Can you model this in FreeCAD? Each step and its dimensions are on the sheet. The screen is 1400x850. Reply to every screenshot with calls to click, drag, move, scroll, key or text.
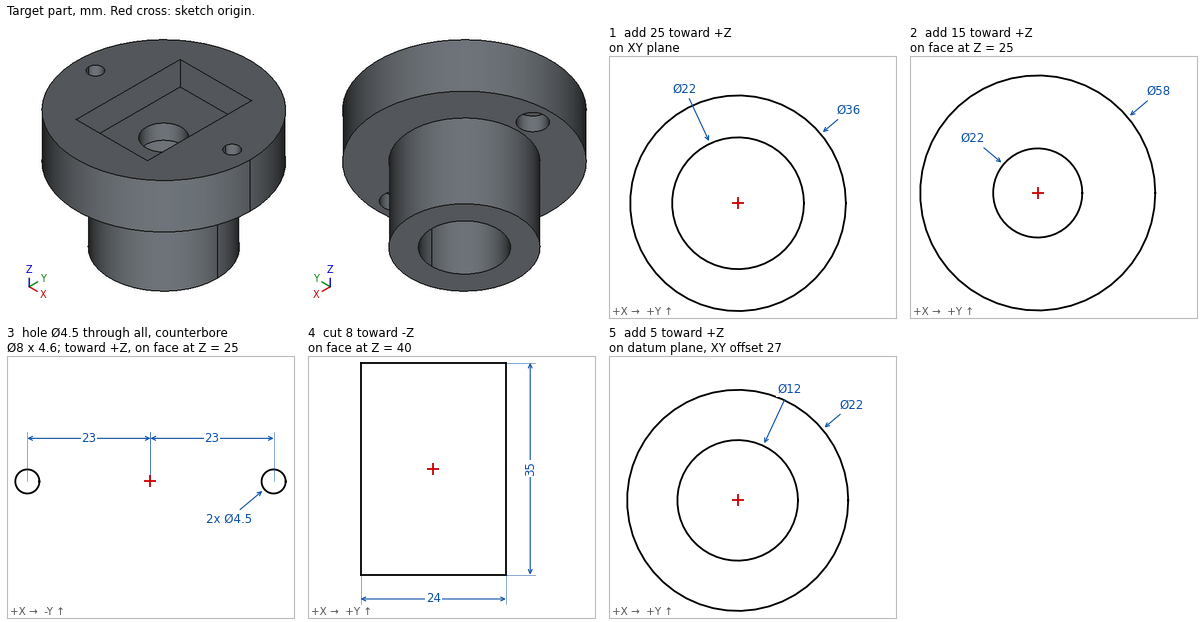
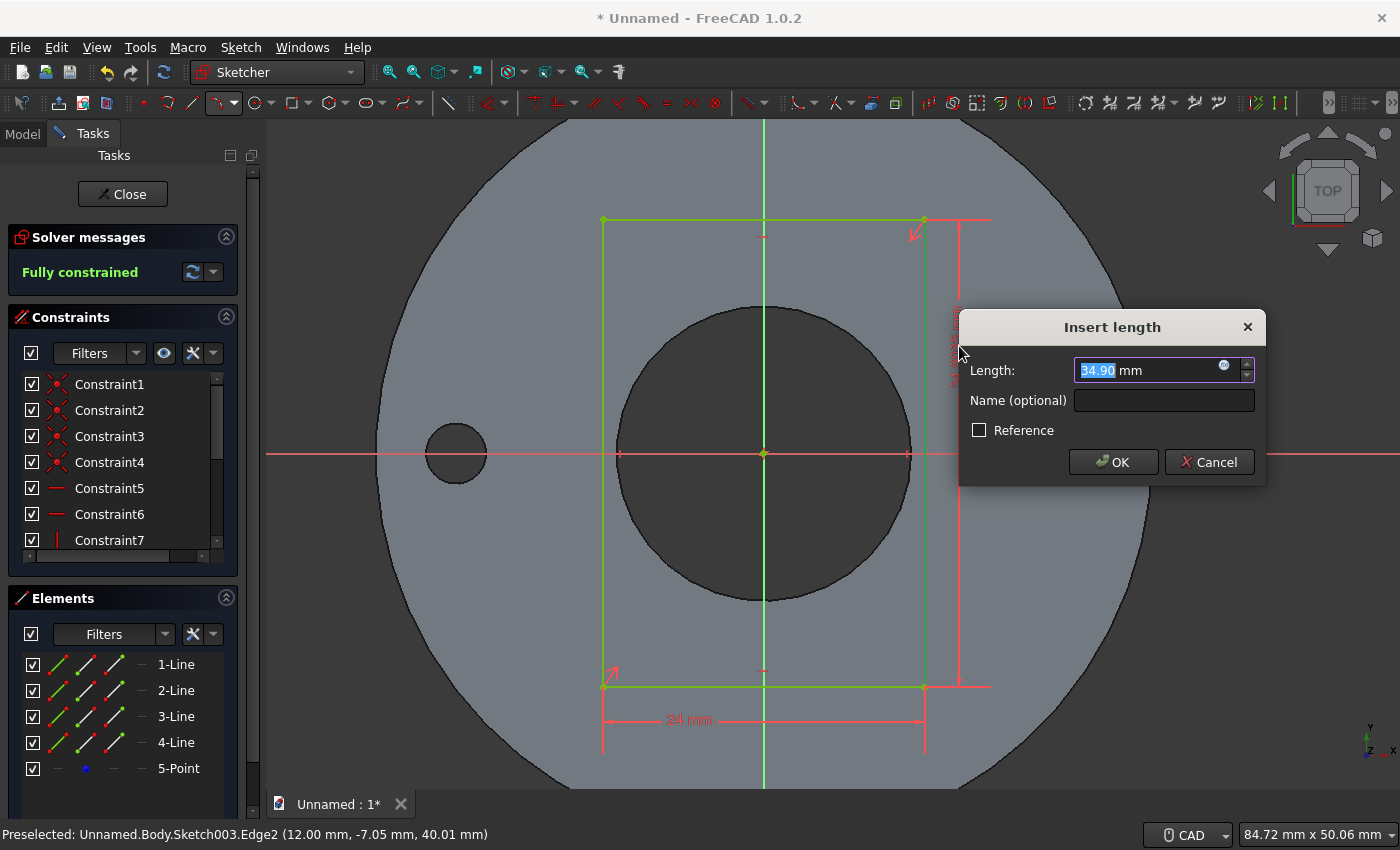
text(35)
key(Return)
key(Escape)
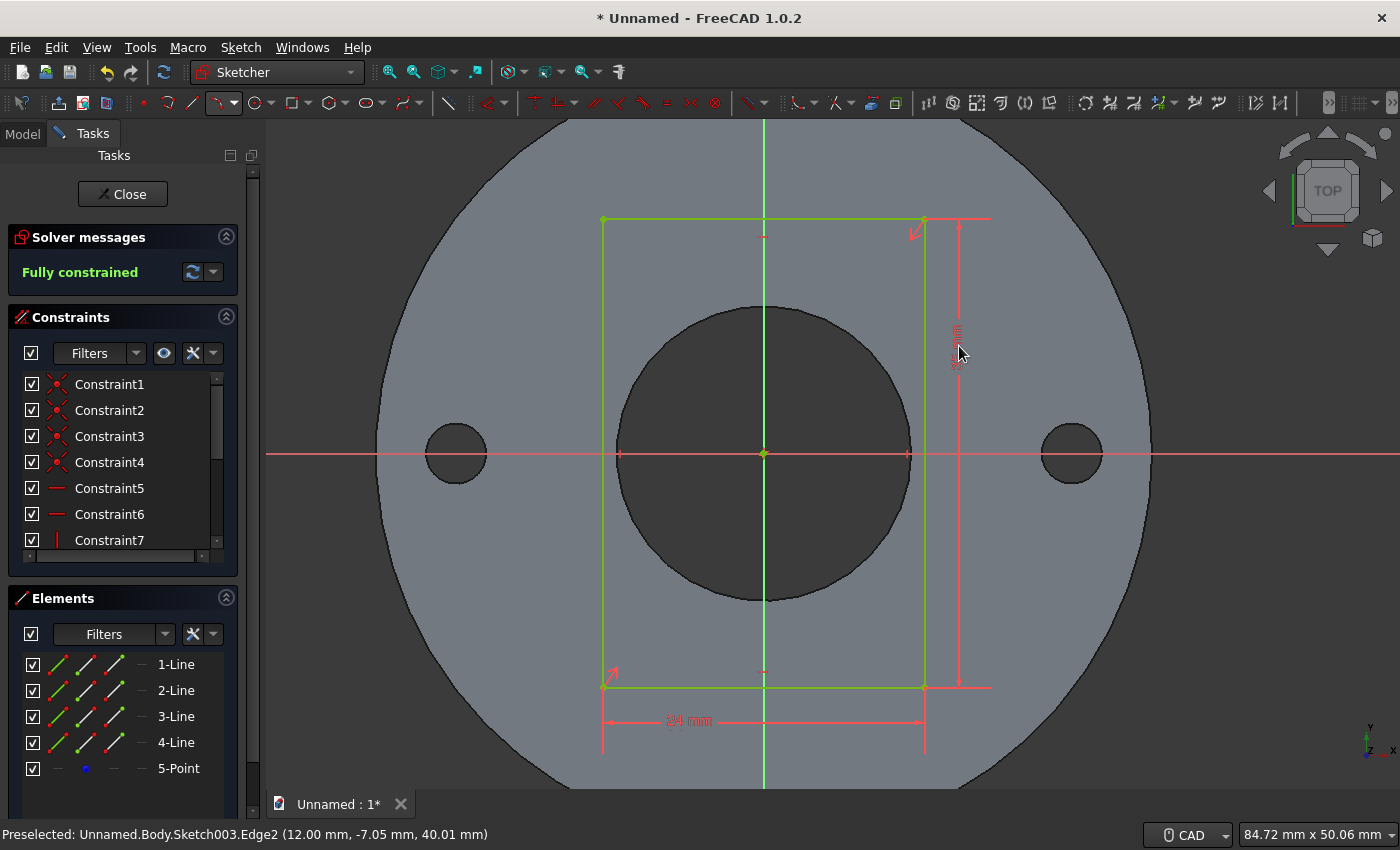
click(123, 194)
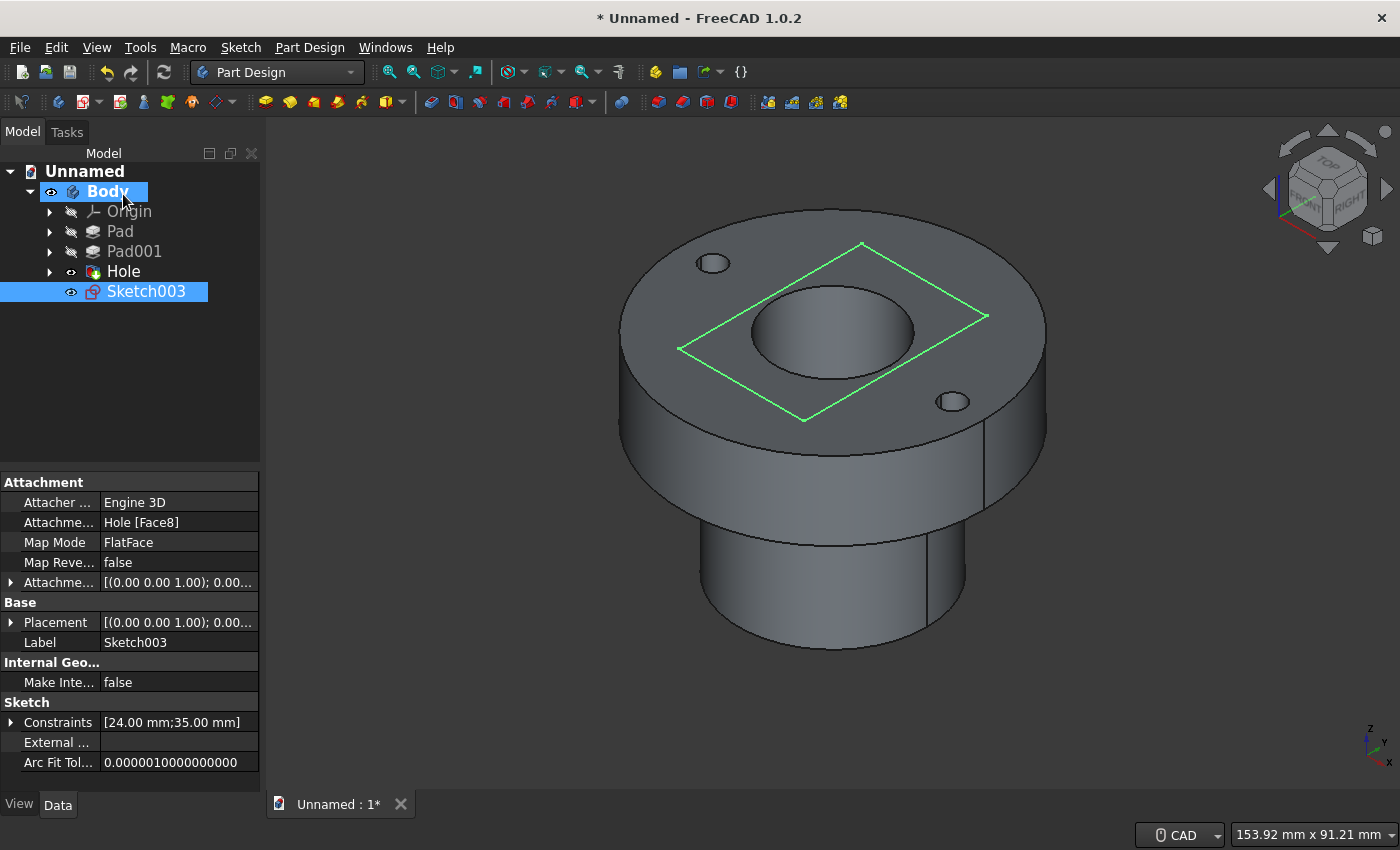
click(432, 102)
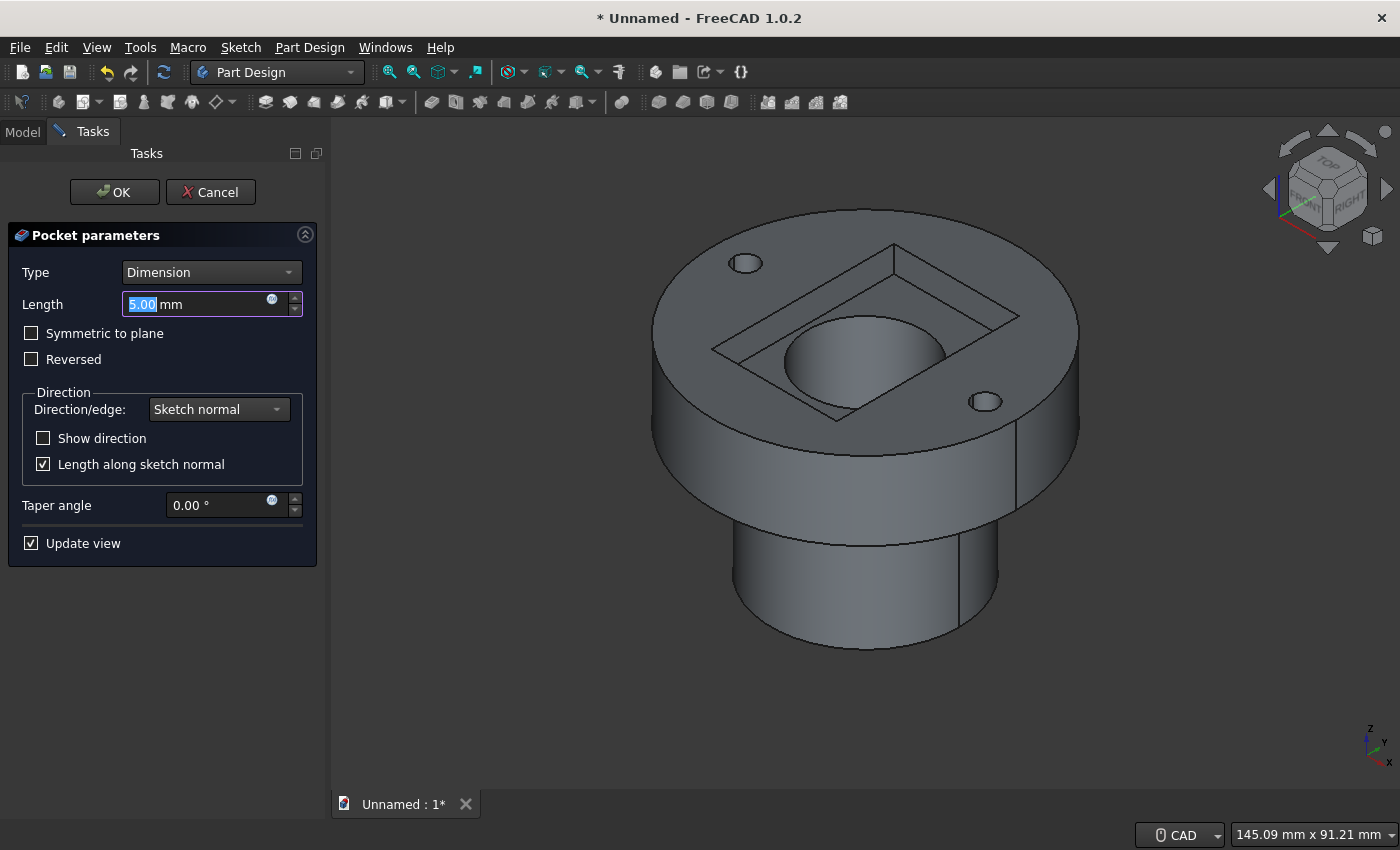
text(8)
key(Tab)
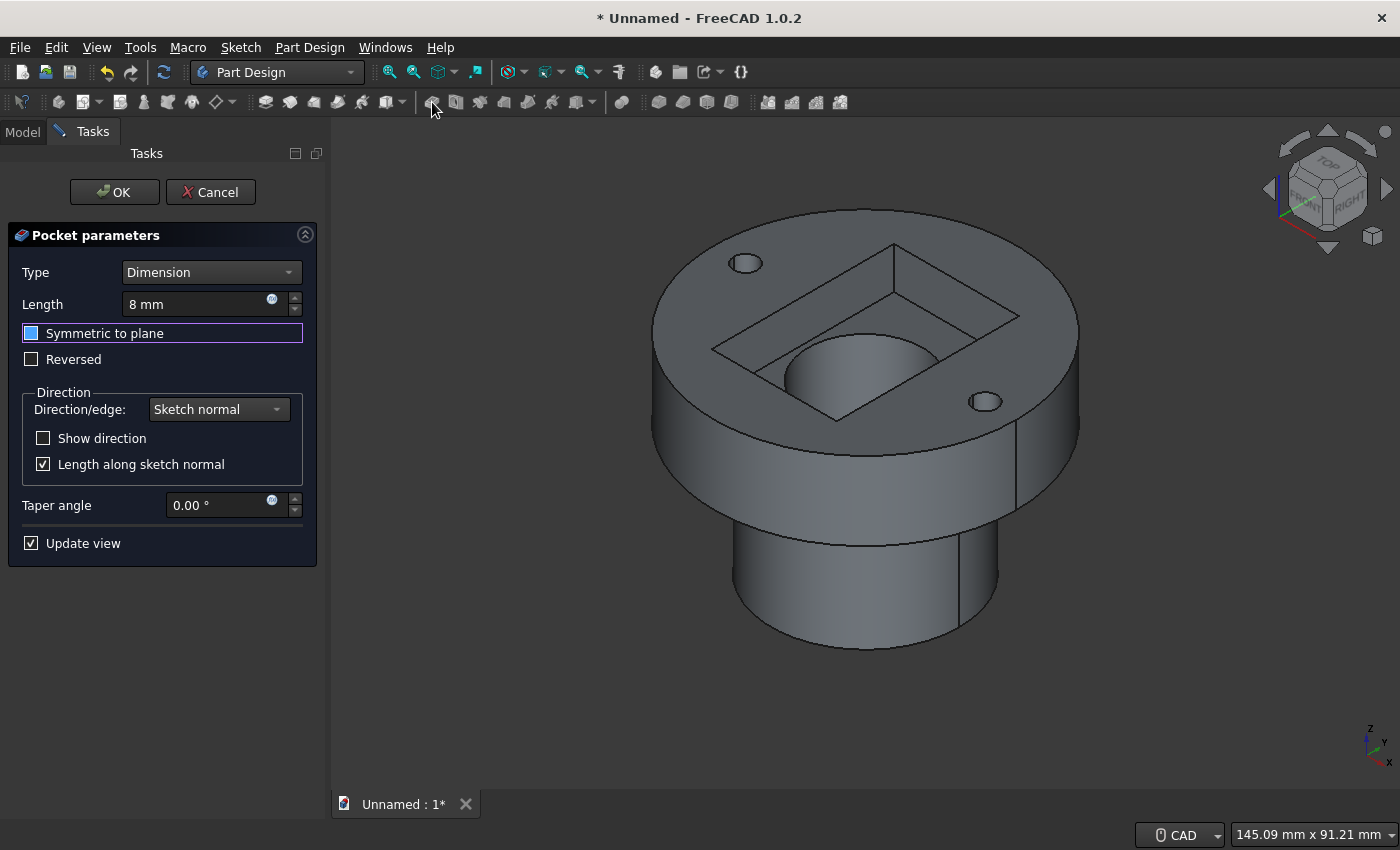
click(115, 192)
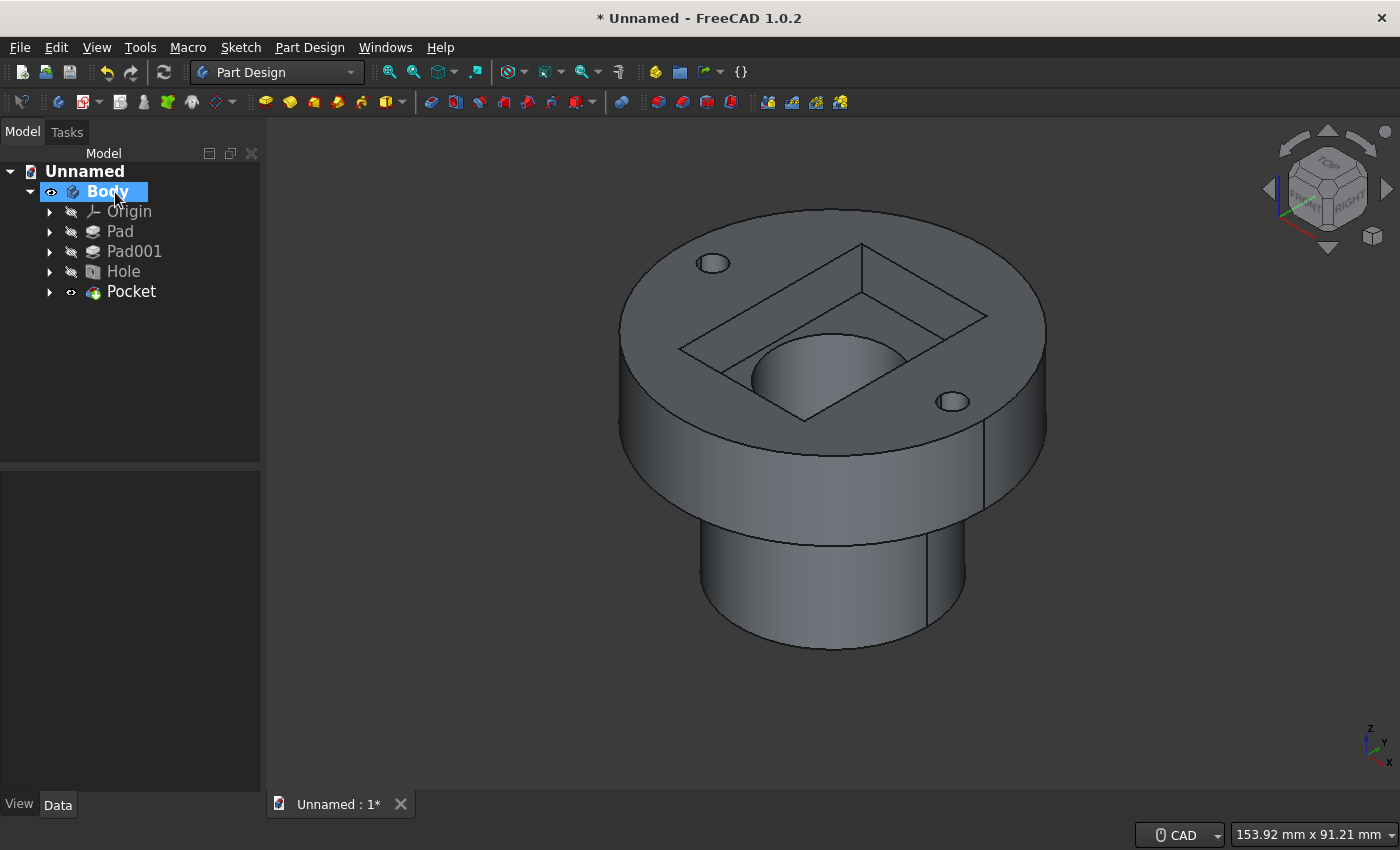
click(50, 212)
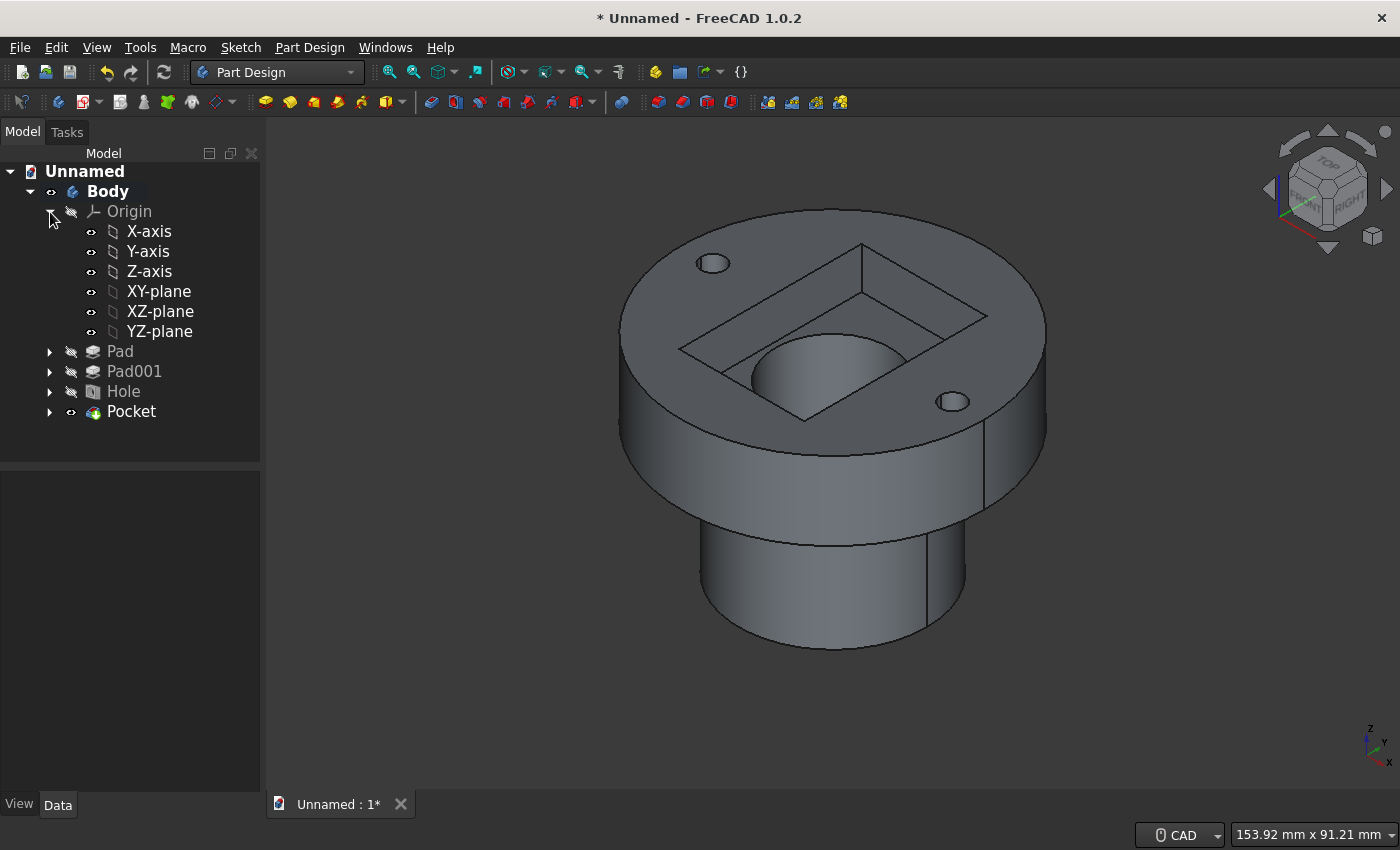
click(136, 292)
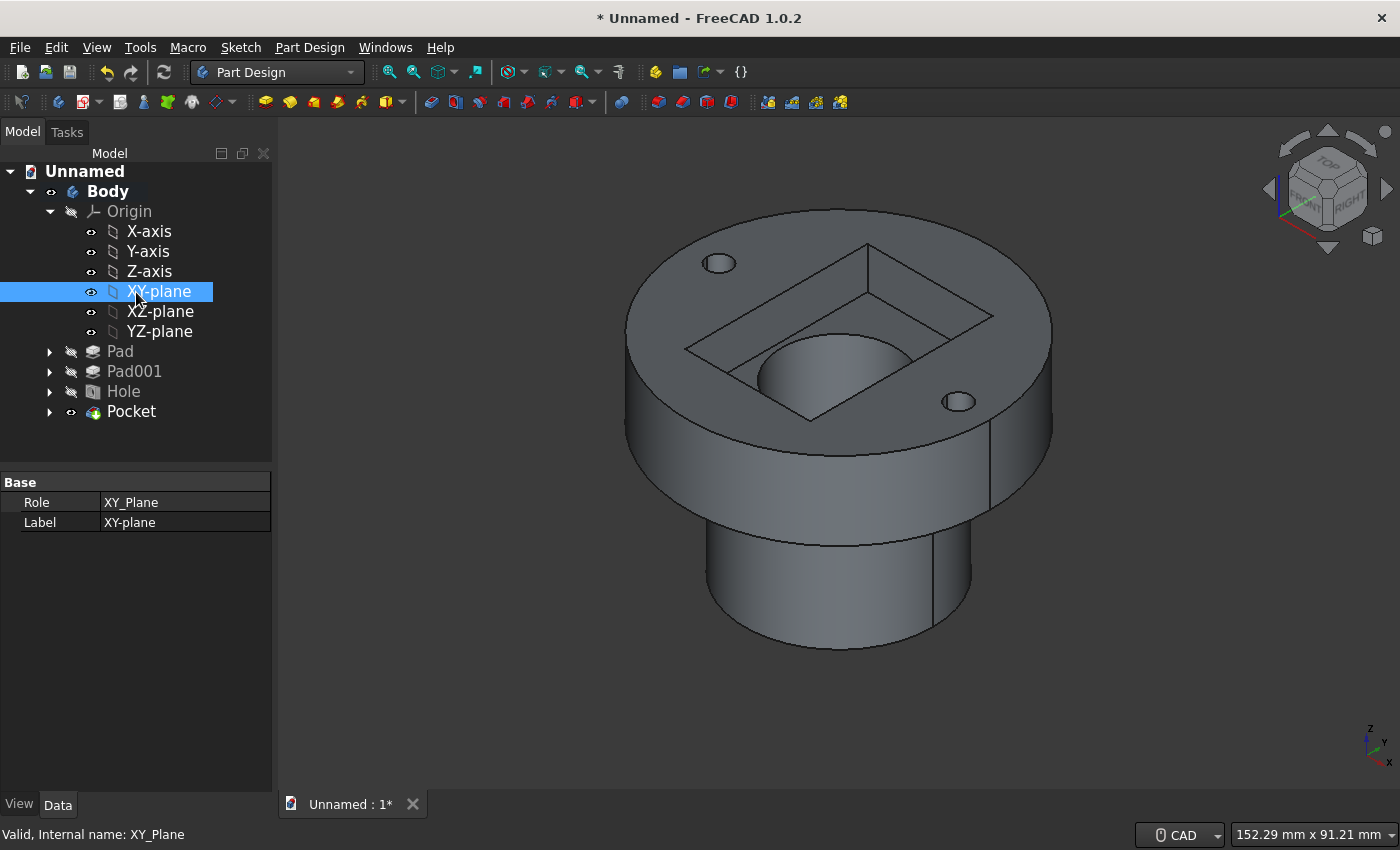
click(216, 102)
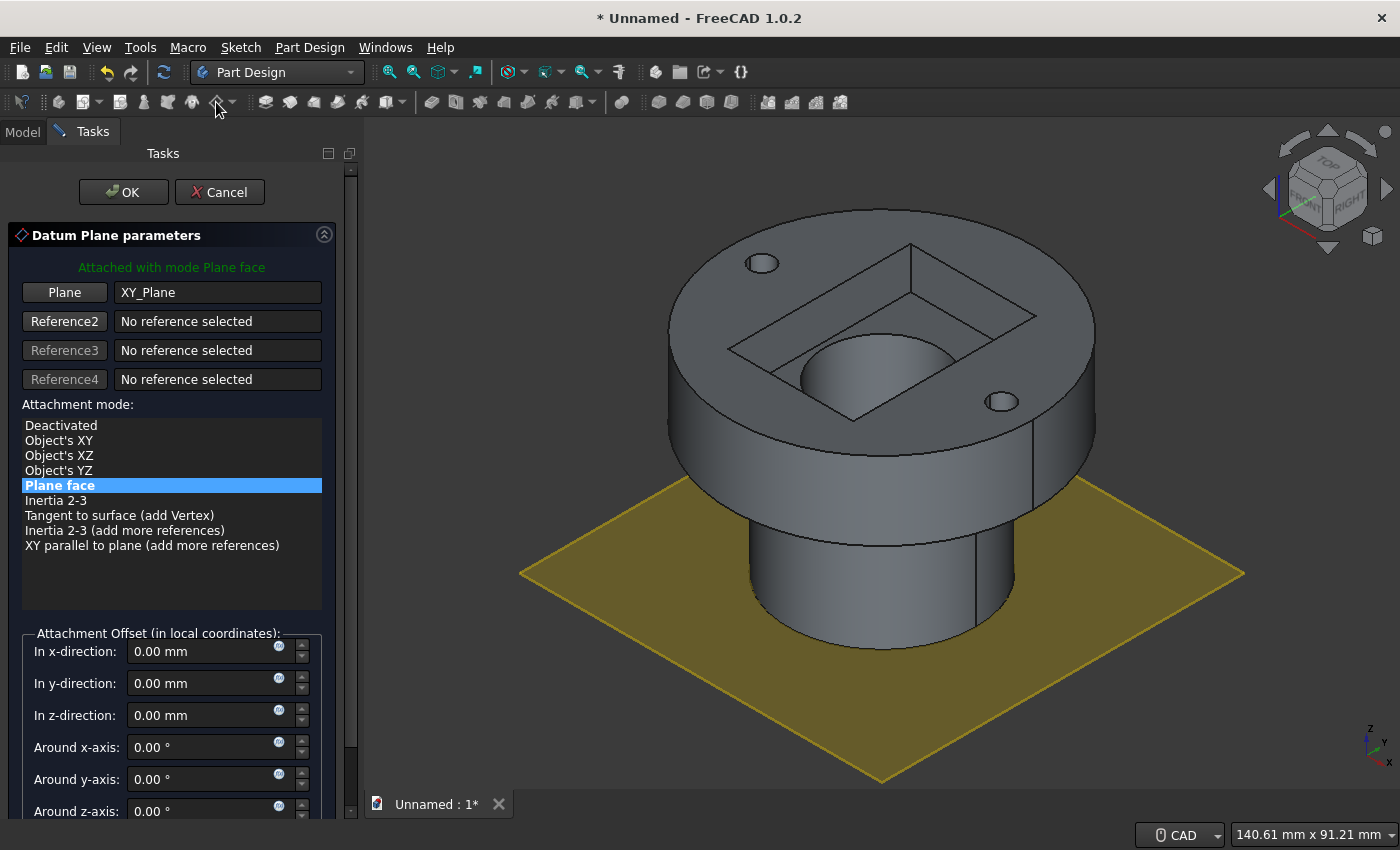
triple_click(210, 715)